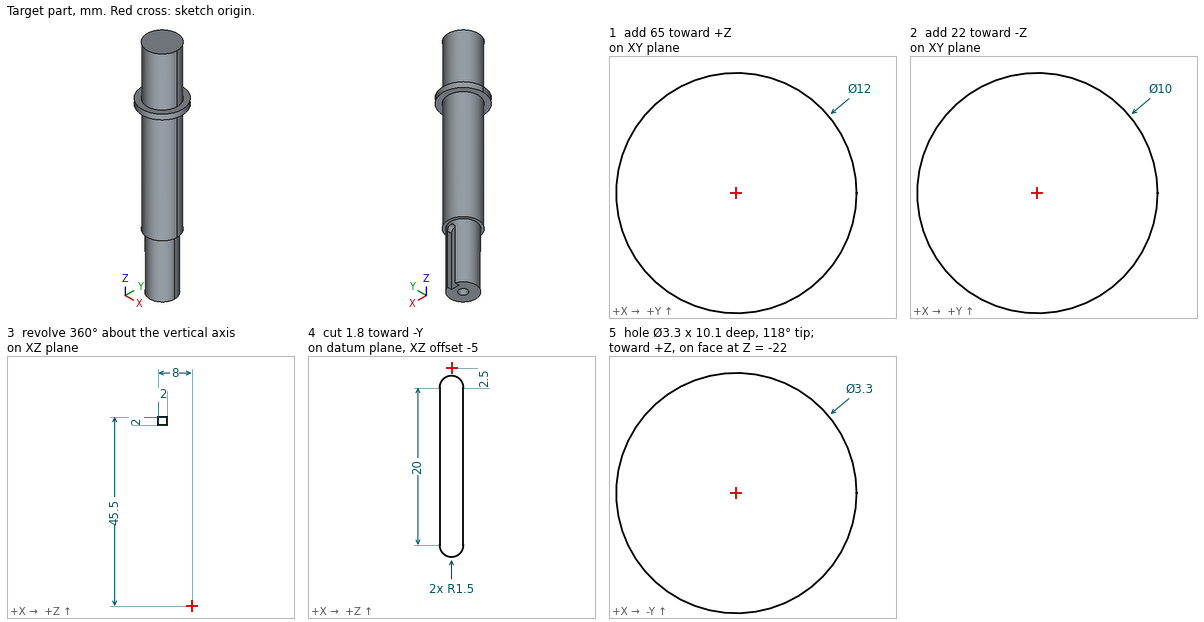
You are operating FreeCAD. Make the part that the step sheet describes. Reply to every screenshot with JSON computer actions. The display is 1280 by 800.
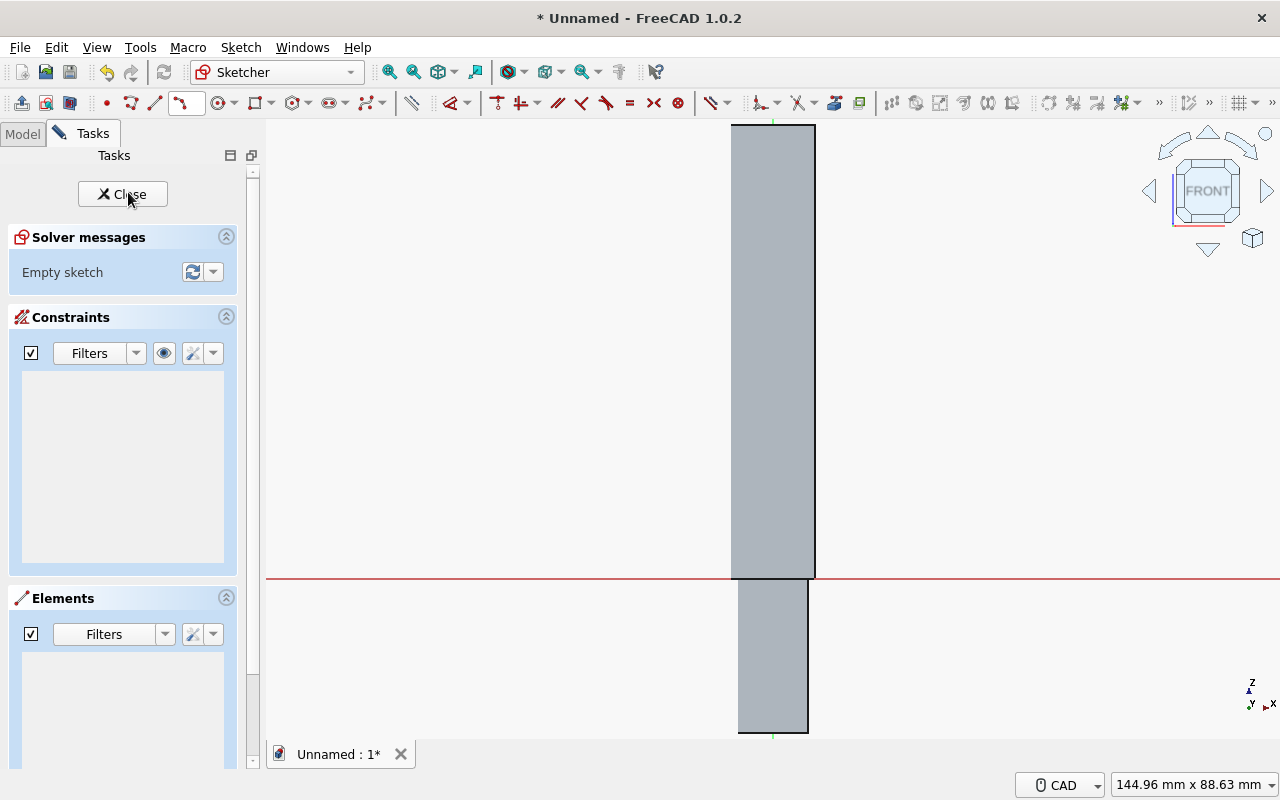
{"action": "left_click", "coordinate": [70, 104]}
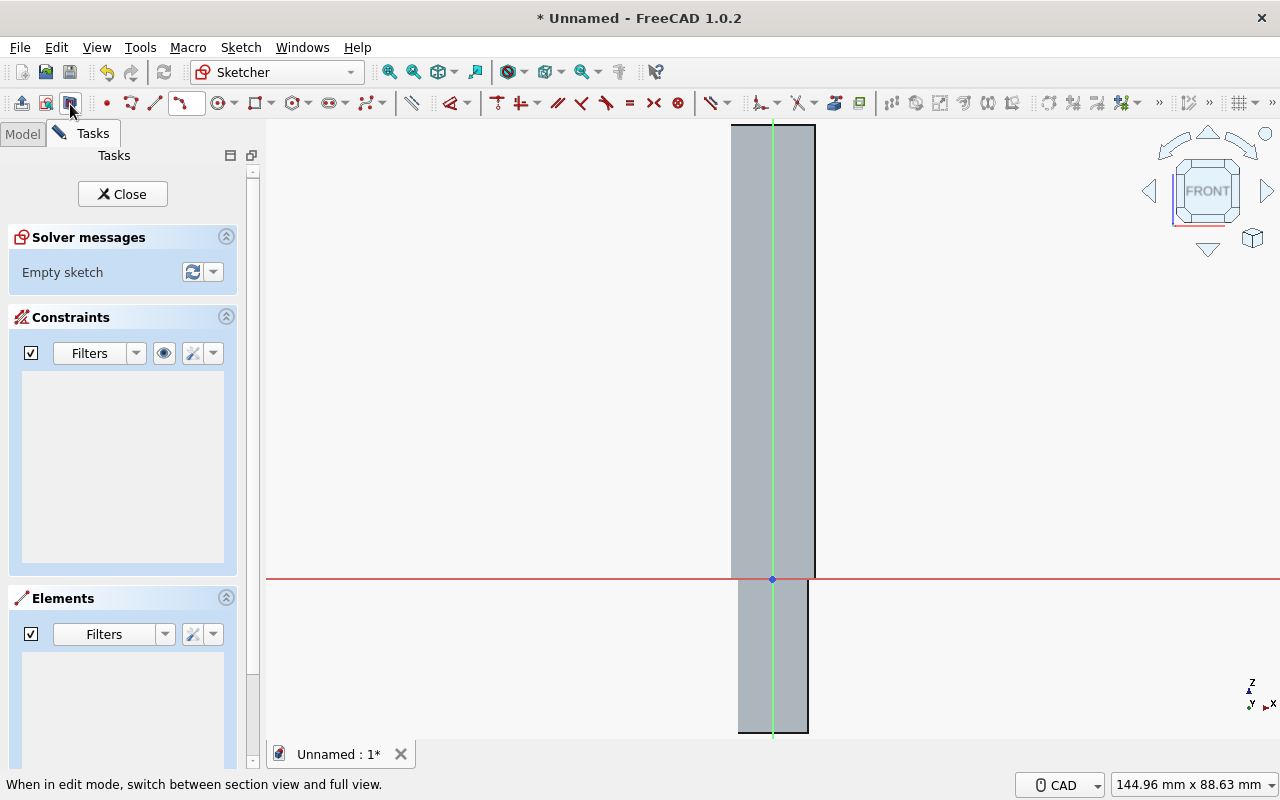
{"action": "scroll", "coordinate": [725, 260], "scroll_direction": "up", "scroll_amount": 15}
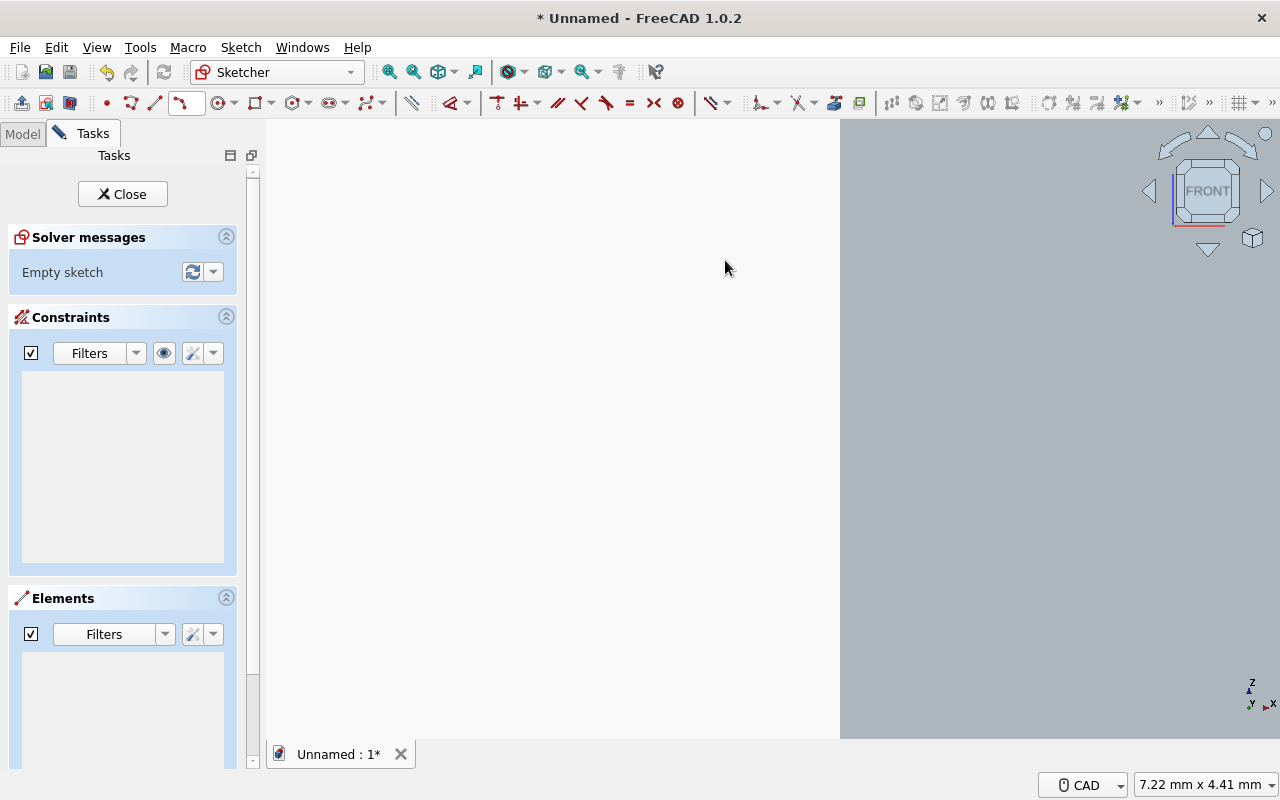
{"action": "scroll", "coordinate": [674, 397], "scroll_direction": "up", "scroll_amount": 2}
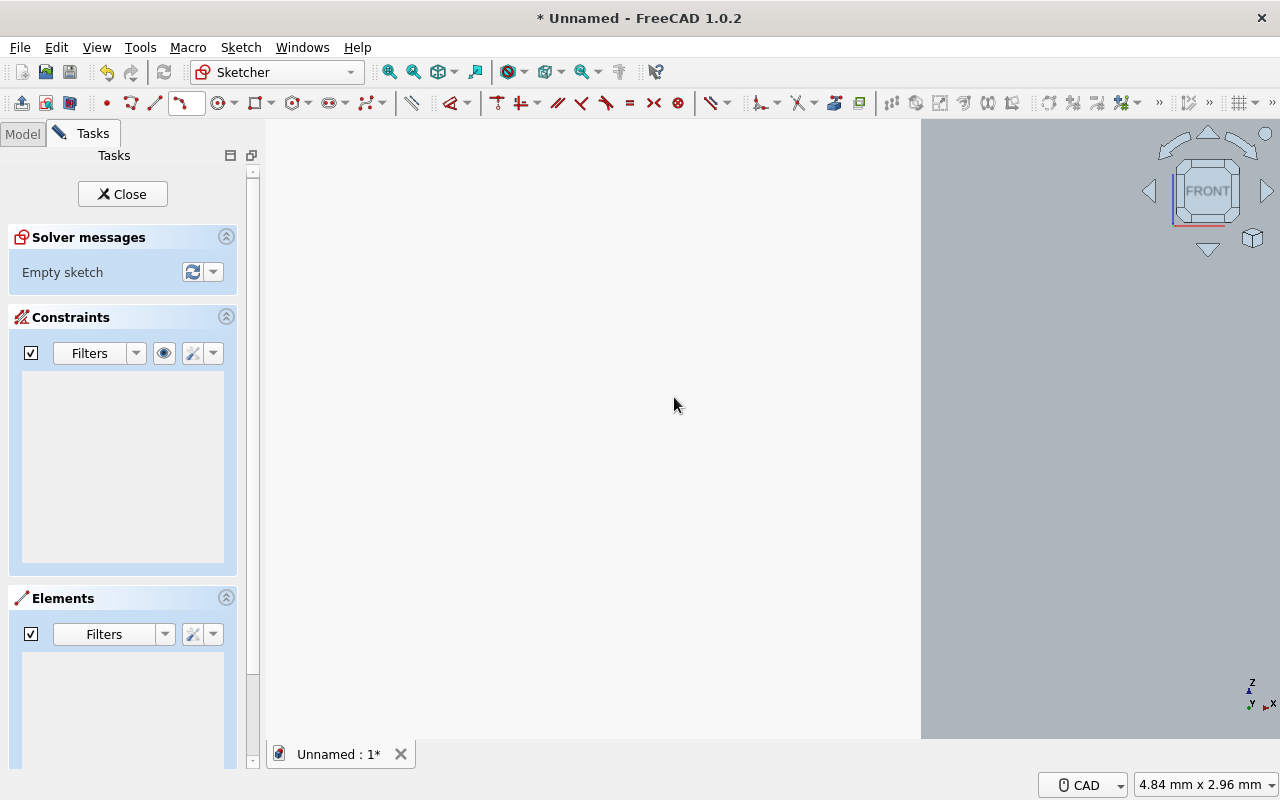
{"action": "left_click", "coordinate": [256, 104]}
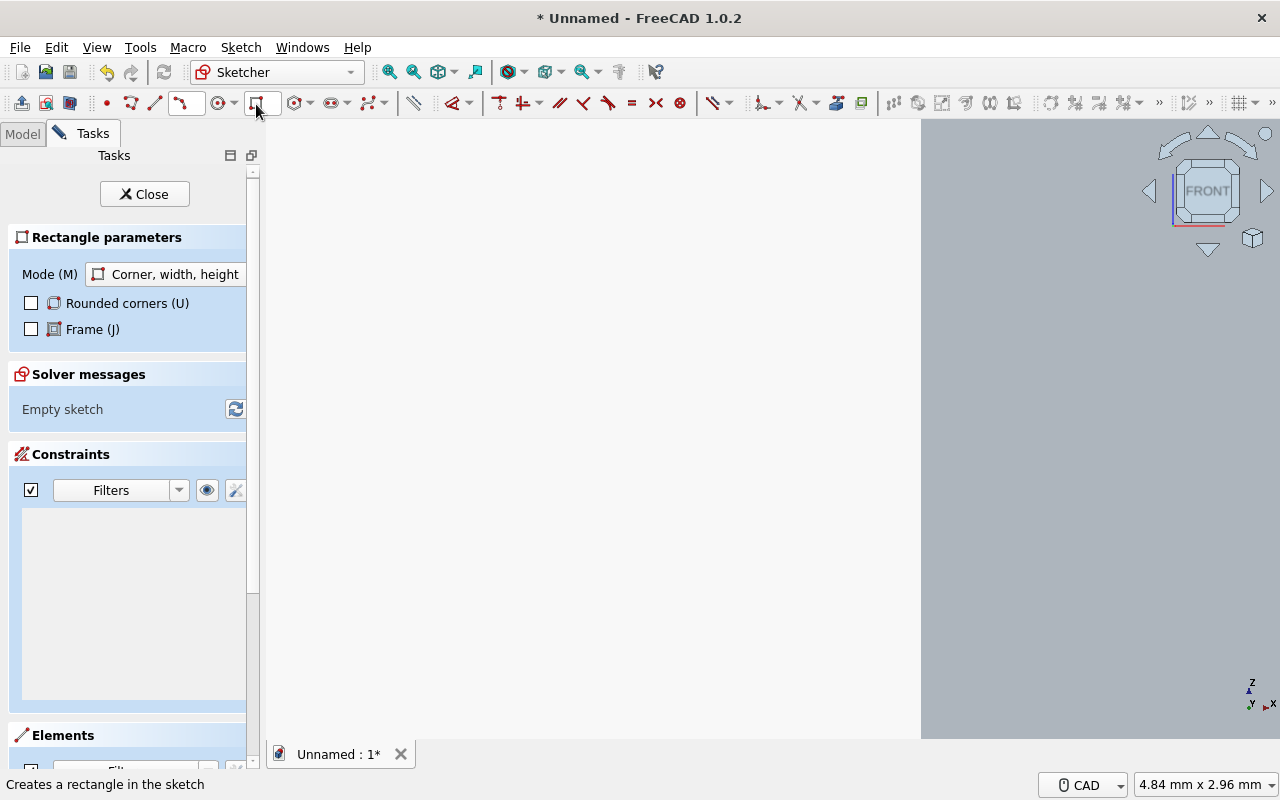
{"action": "left_click", "coordinate": [495, 219]}
{"action": "mouse_move", "coordinate": [914, 639]}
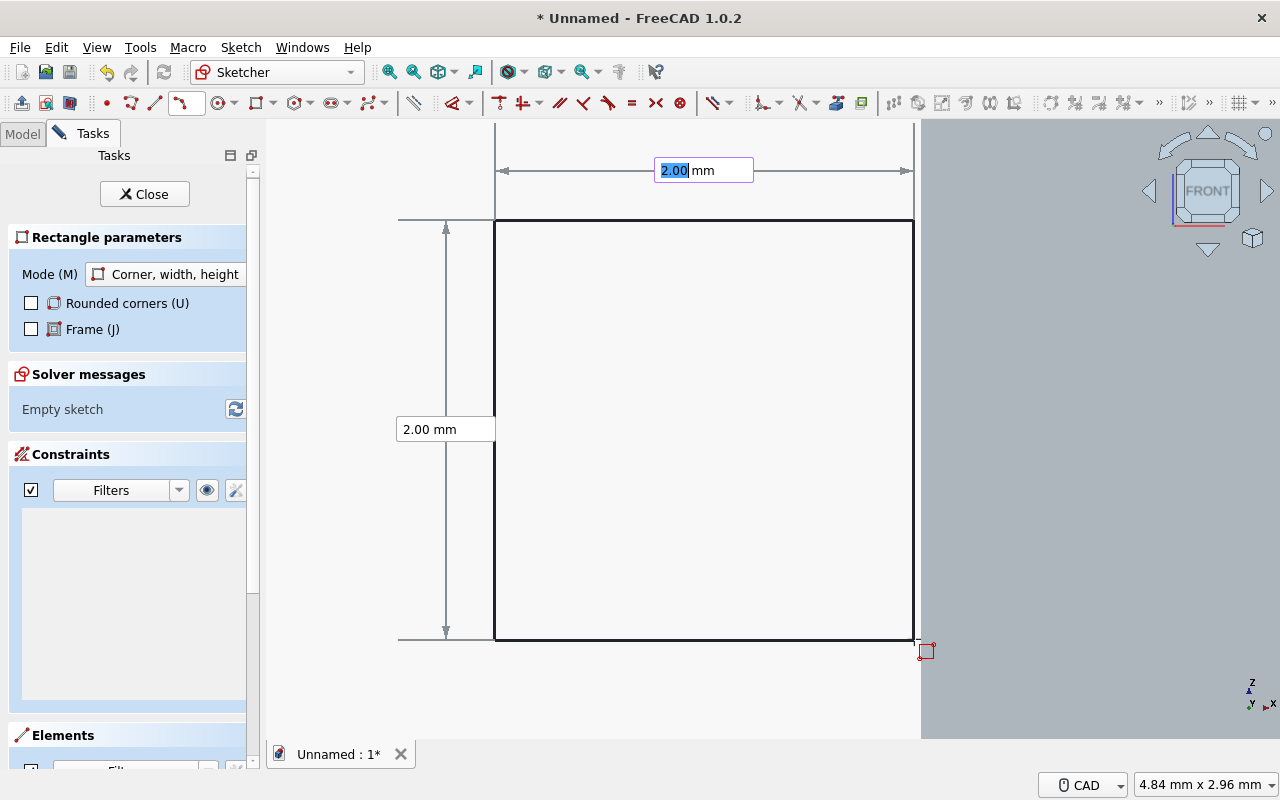
{"action": "type", "text": "2"}
{"action": "key", "text": "Tab"}
{"action": "type", "text": "2"}
{"action": "key", "text": "Return"}
{"action": "key", "text": "Escape"}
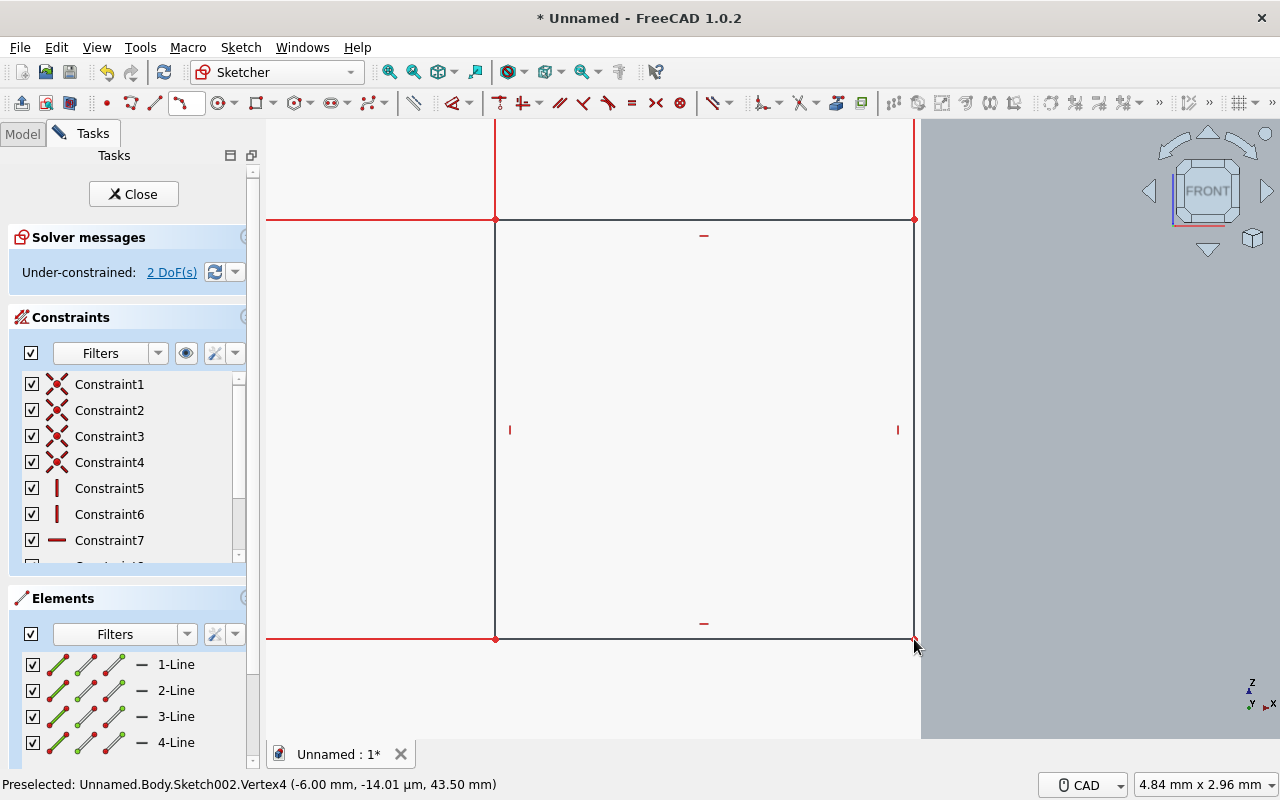
{"action": "left_click", "coordinate": [452, 104]}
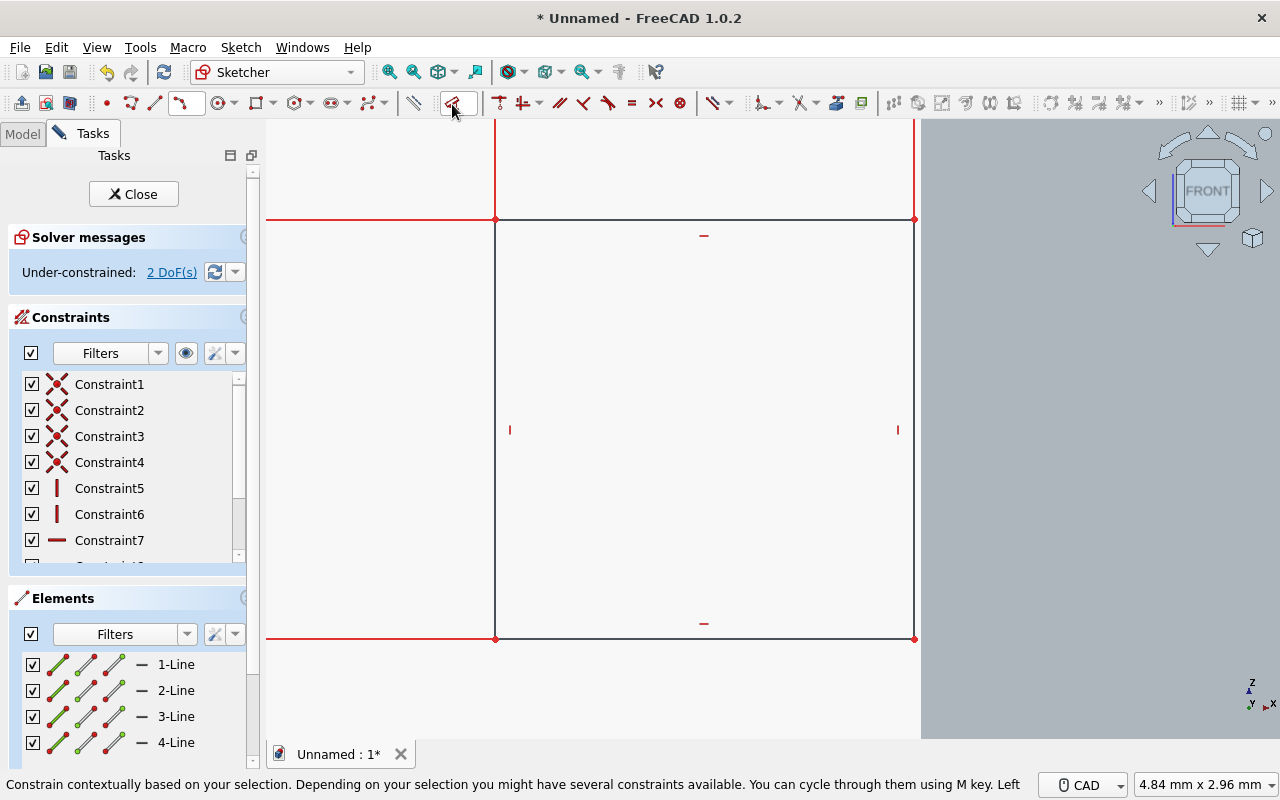
{"action": "left_click", "coordinate": [495, 220]}
{"action": "left_click", "coordinate": [805, 186]}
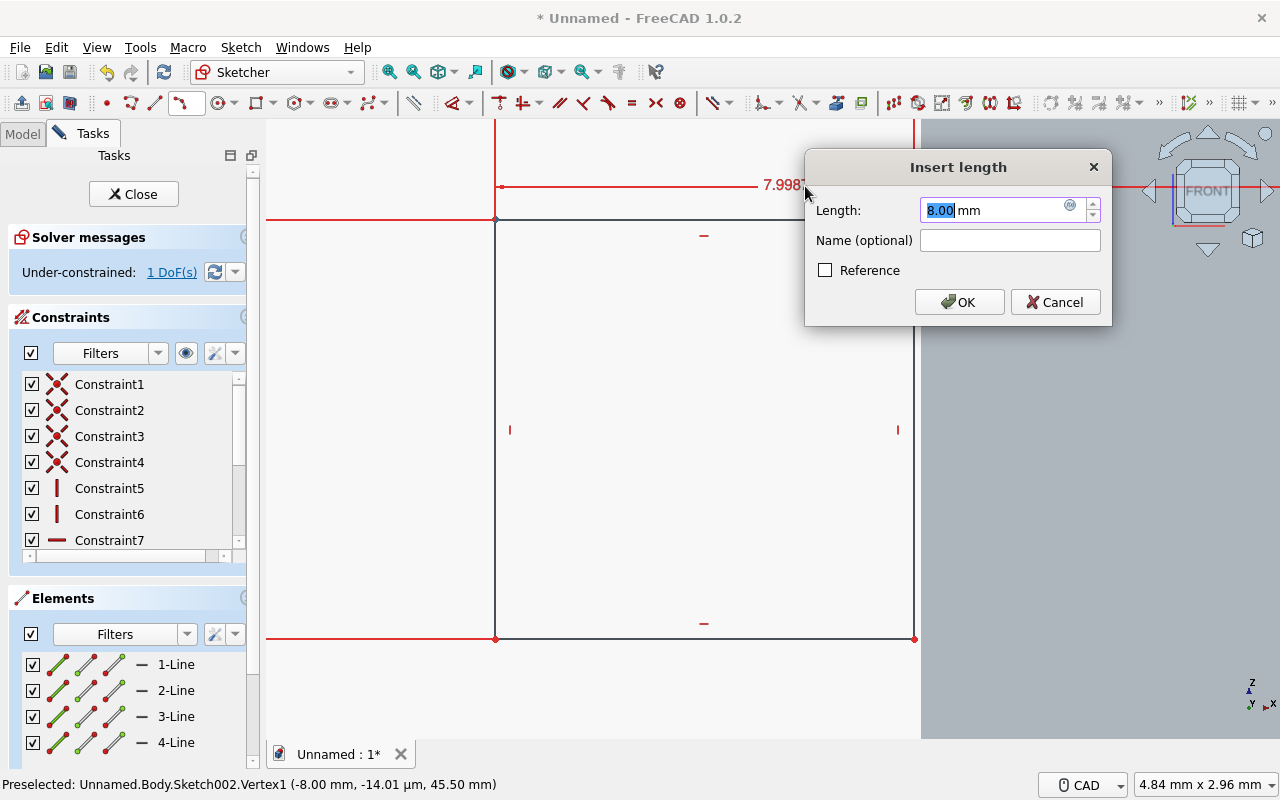
{"action": "type", "text": "8"}
{"action": "key", "text": "Return"}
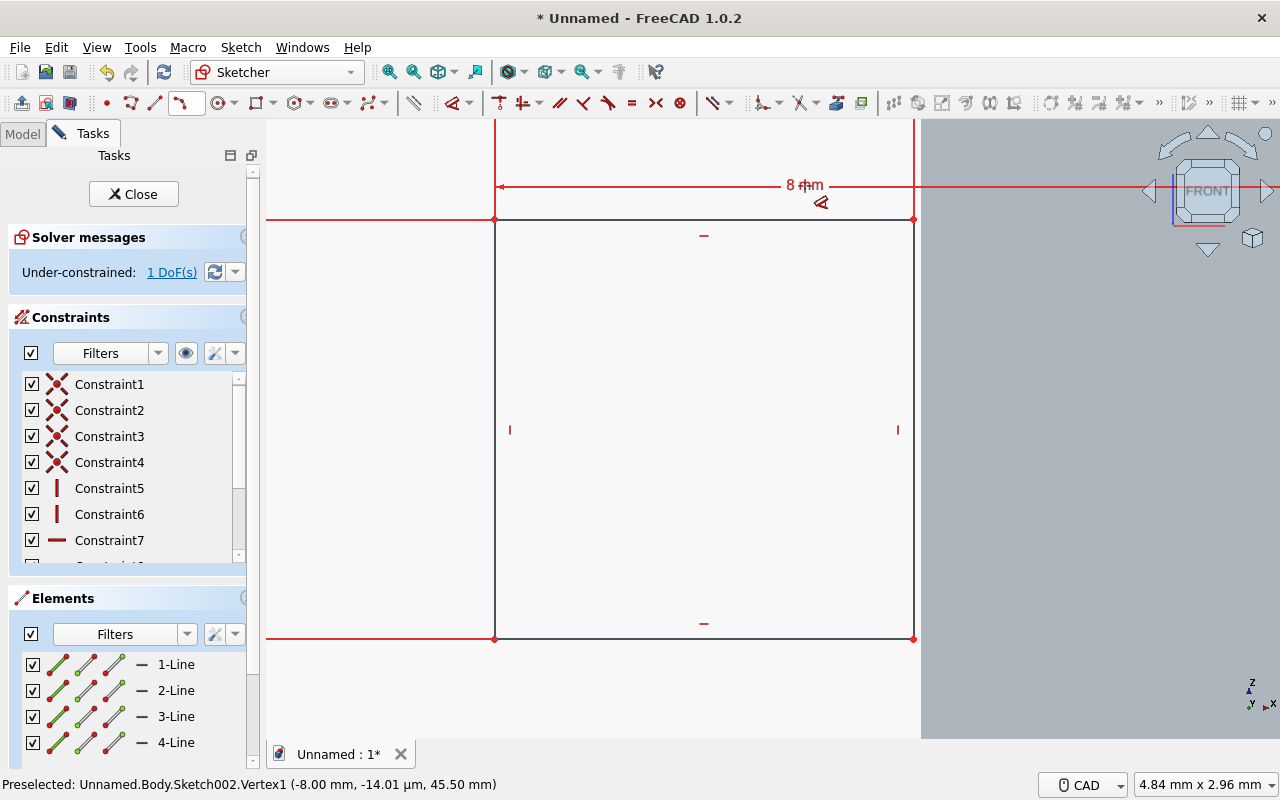
{"action": "left_click", "coordinate": [495, 220]}
{"action": "left_click", "coordinate": [461, 465]}